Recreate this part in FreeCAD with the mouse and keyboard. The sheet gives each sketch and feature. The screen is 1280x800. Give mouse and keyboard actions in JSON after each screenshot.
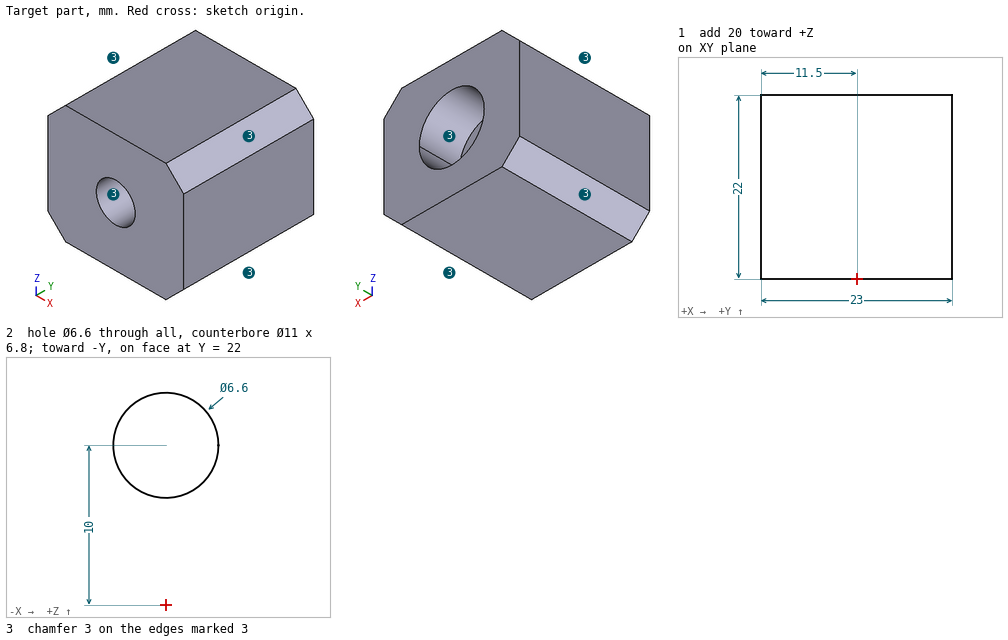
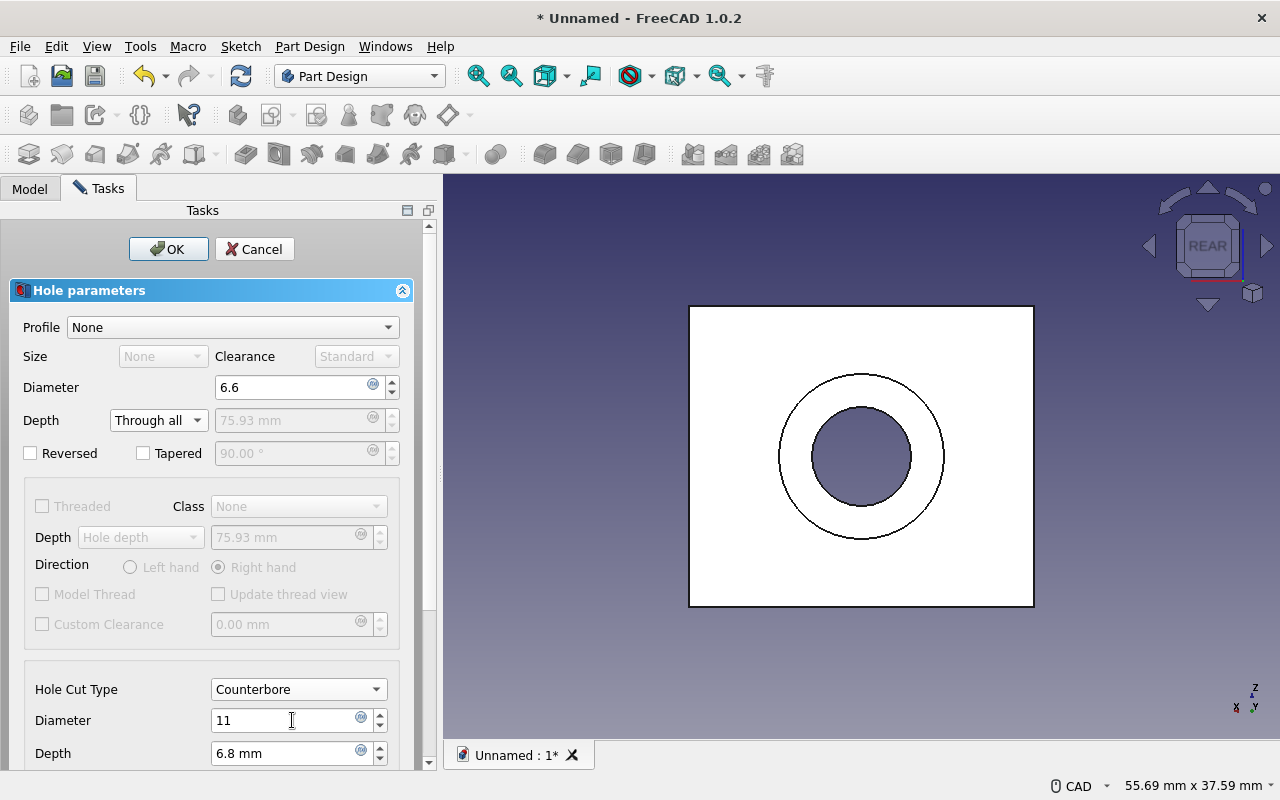
{"action": "left_click", "coordinate": [169, 249]}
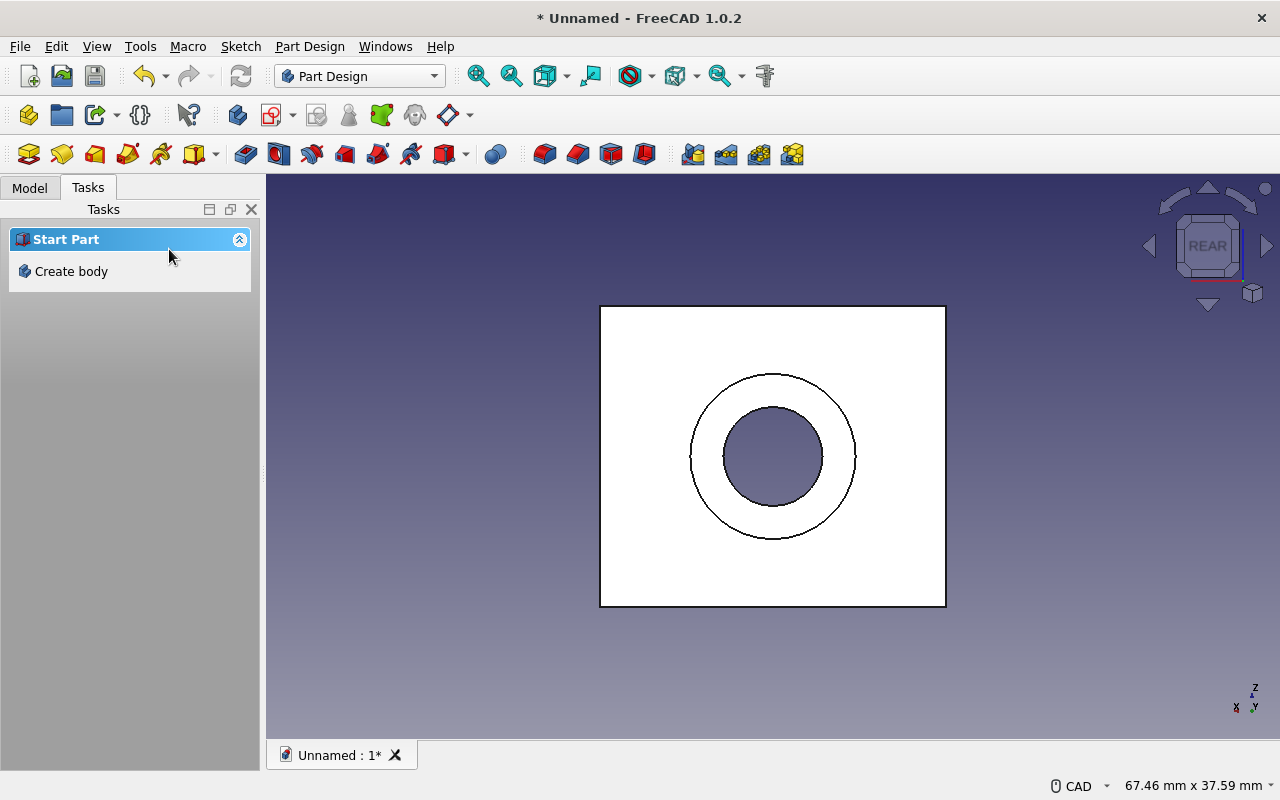
{"action": "key", "text": "0"}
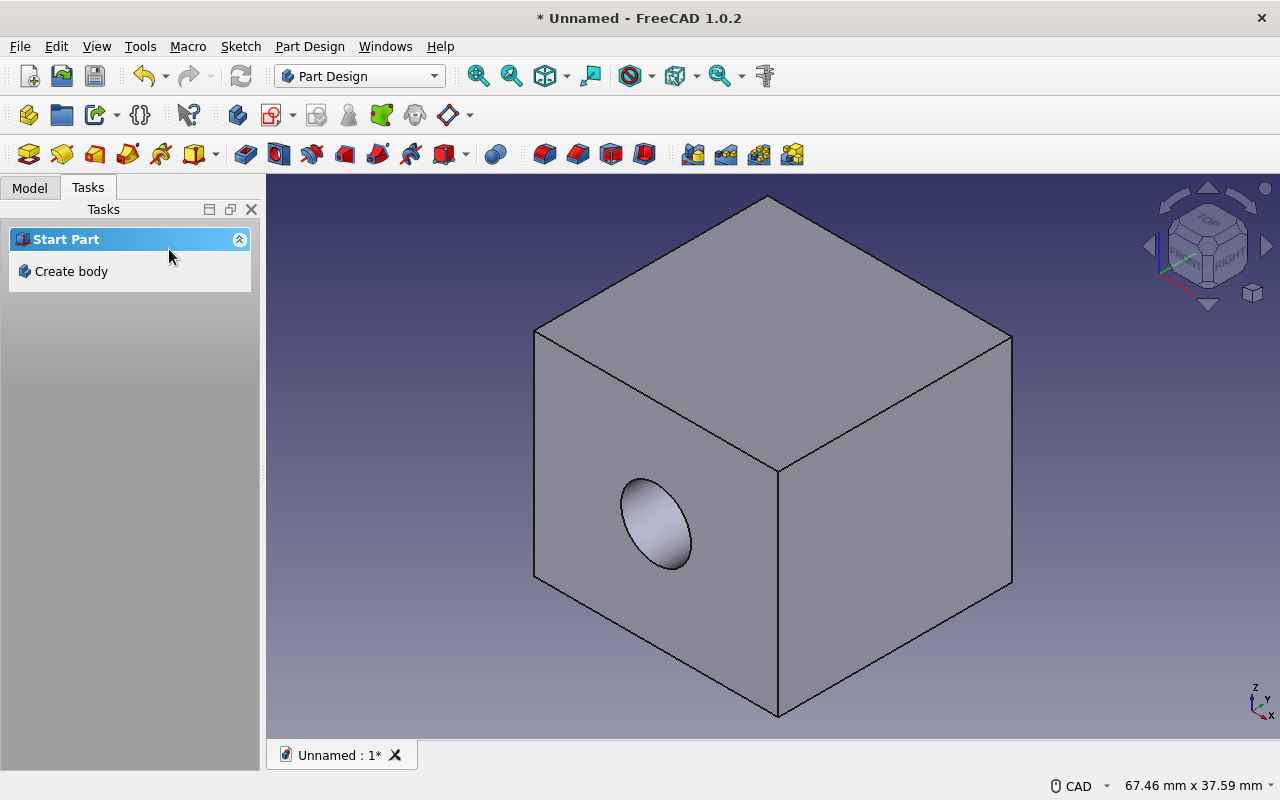
{"action": "left_click", "coordinate": [895, 403]}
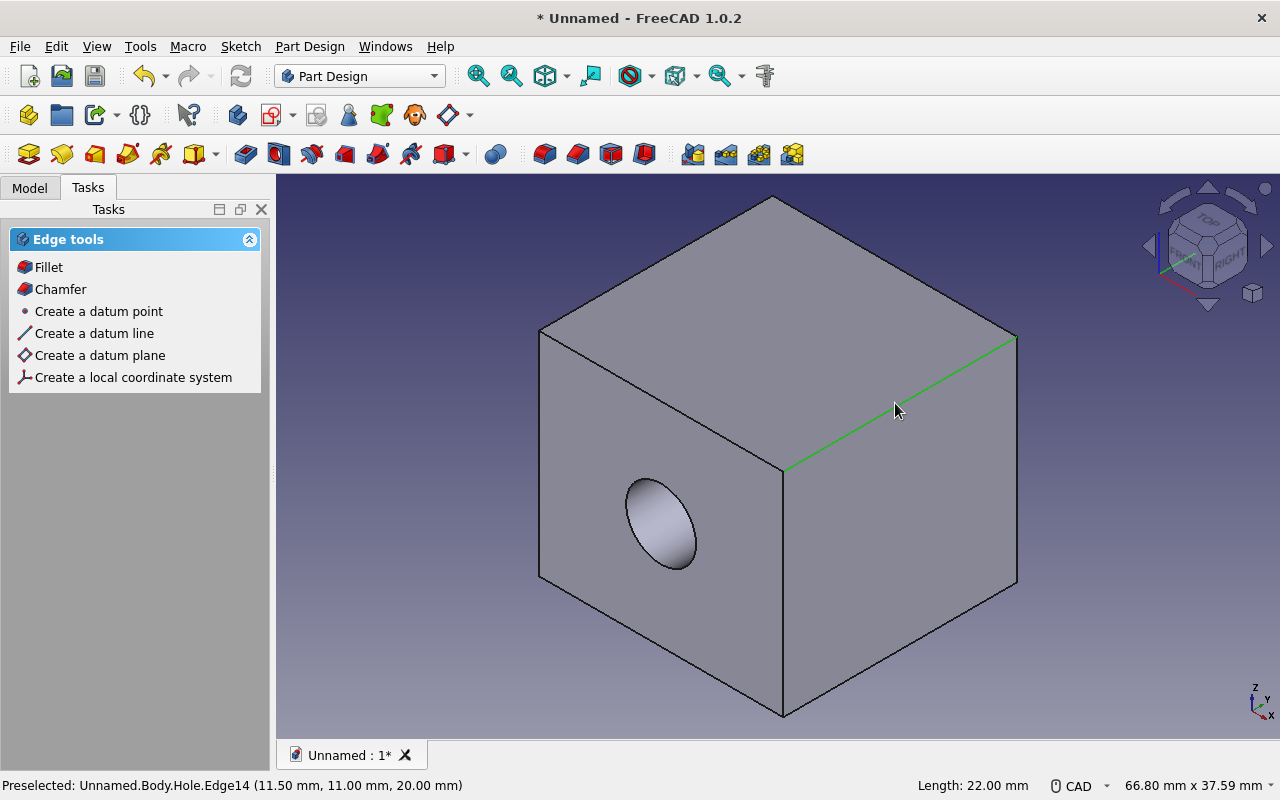
{"action": "key", "text": "2"}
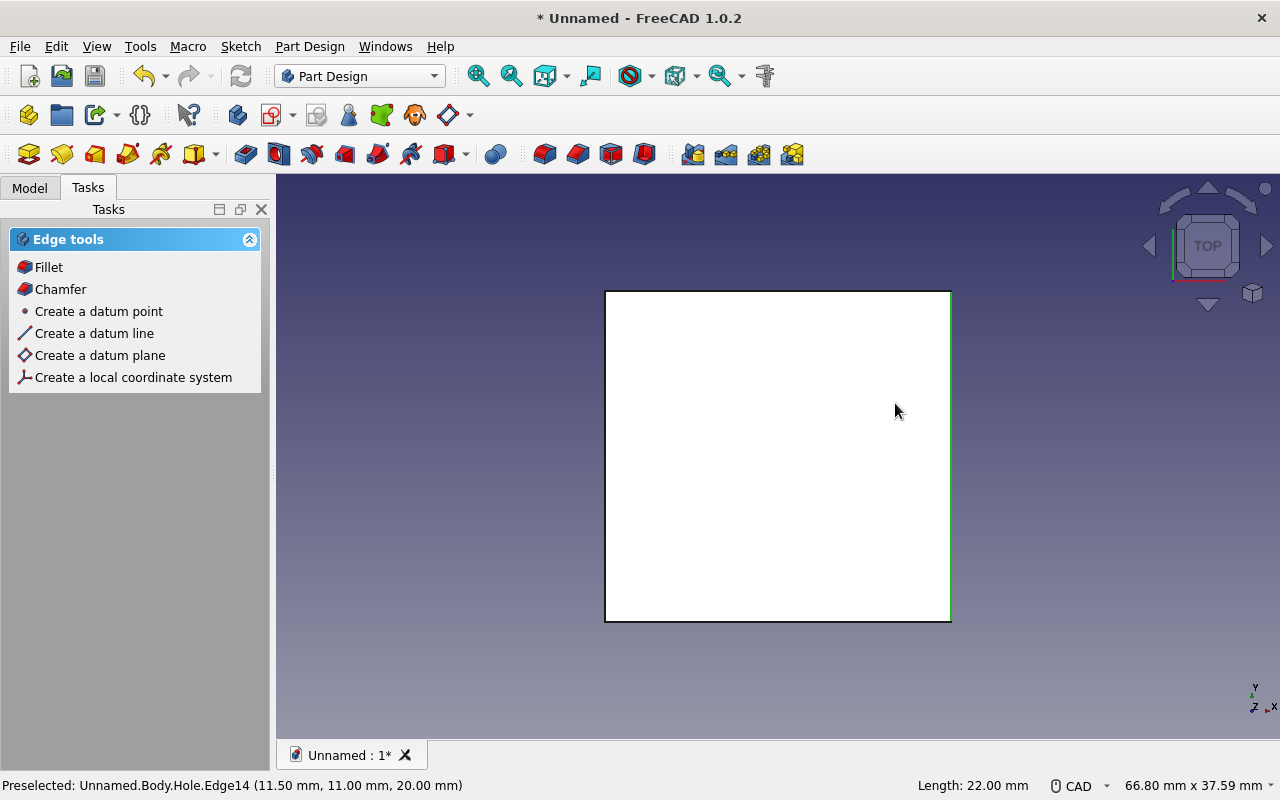
{"action": "left_click", "coordinate": [605, 455], "text": "ctrl"}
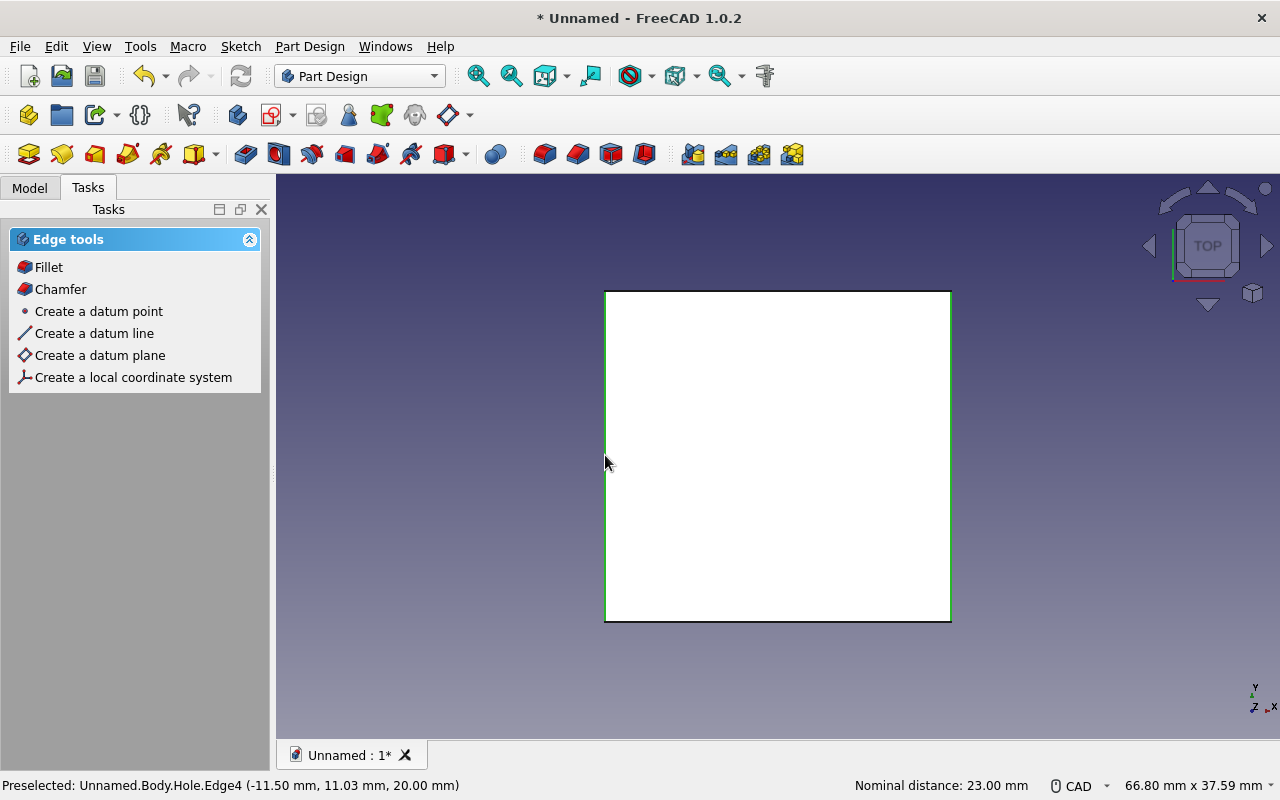
{"action": "key", "text": "1"}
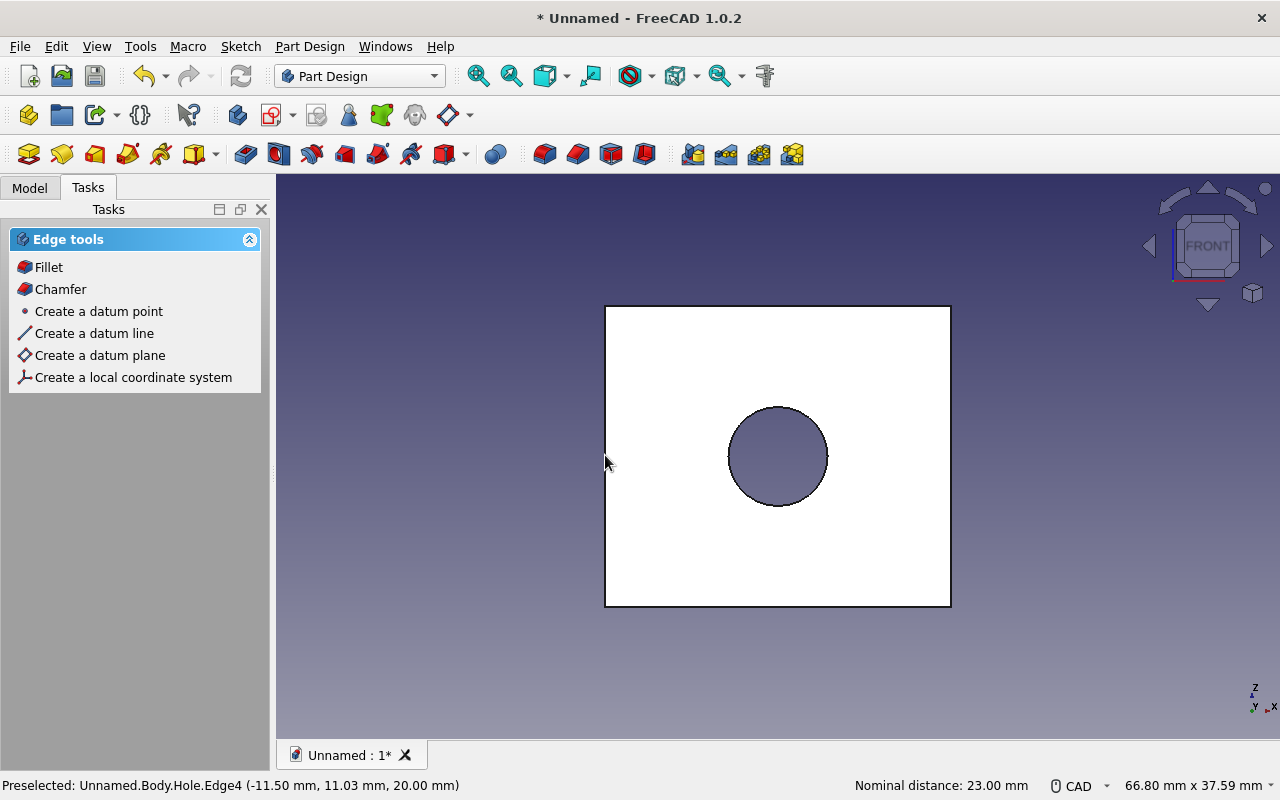
{"action": "key", "text": "3"}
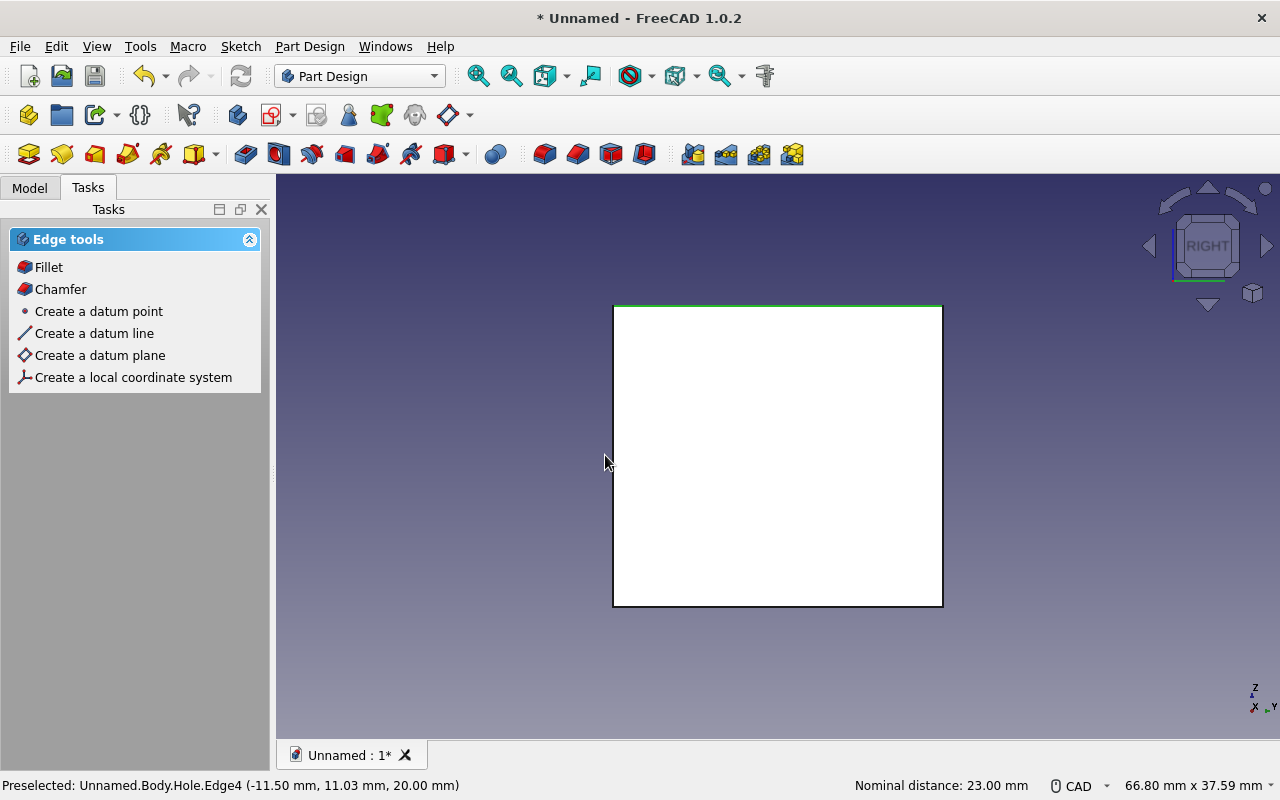
{"action": "left_click", "coordinate": [778, 606], "text": "ctrl"}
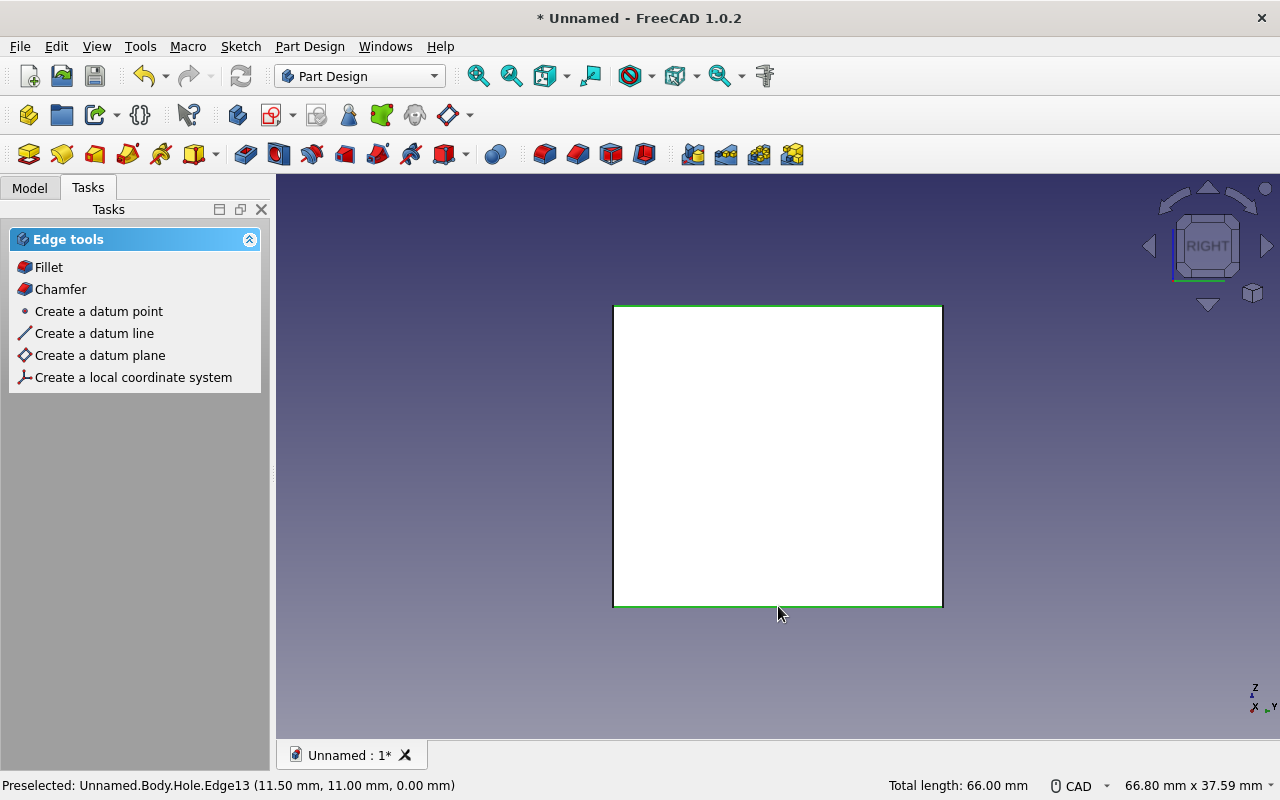
{"action": "key", "text": "5"}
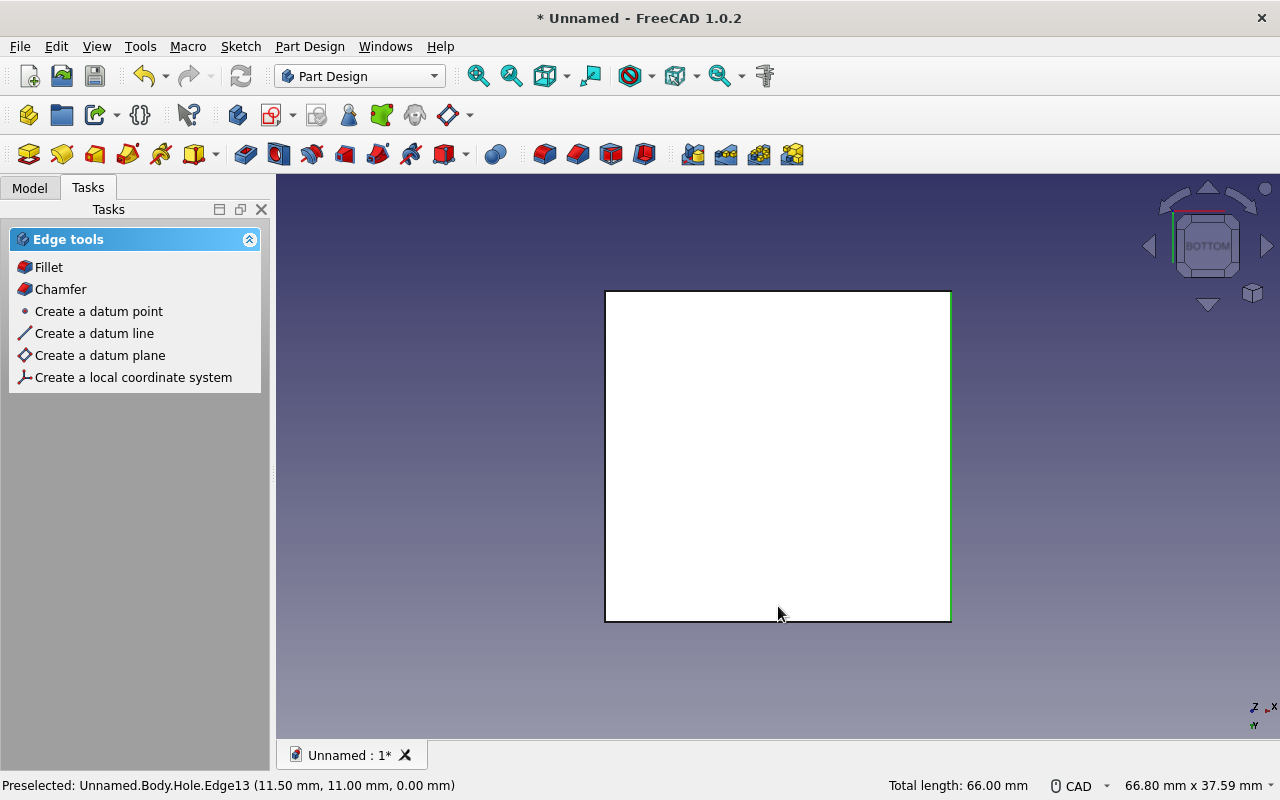
{"action": "left_click", "coordinate": [605, 456], "text": "ctrl"}